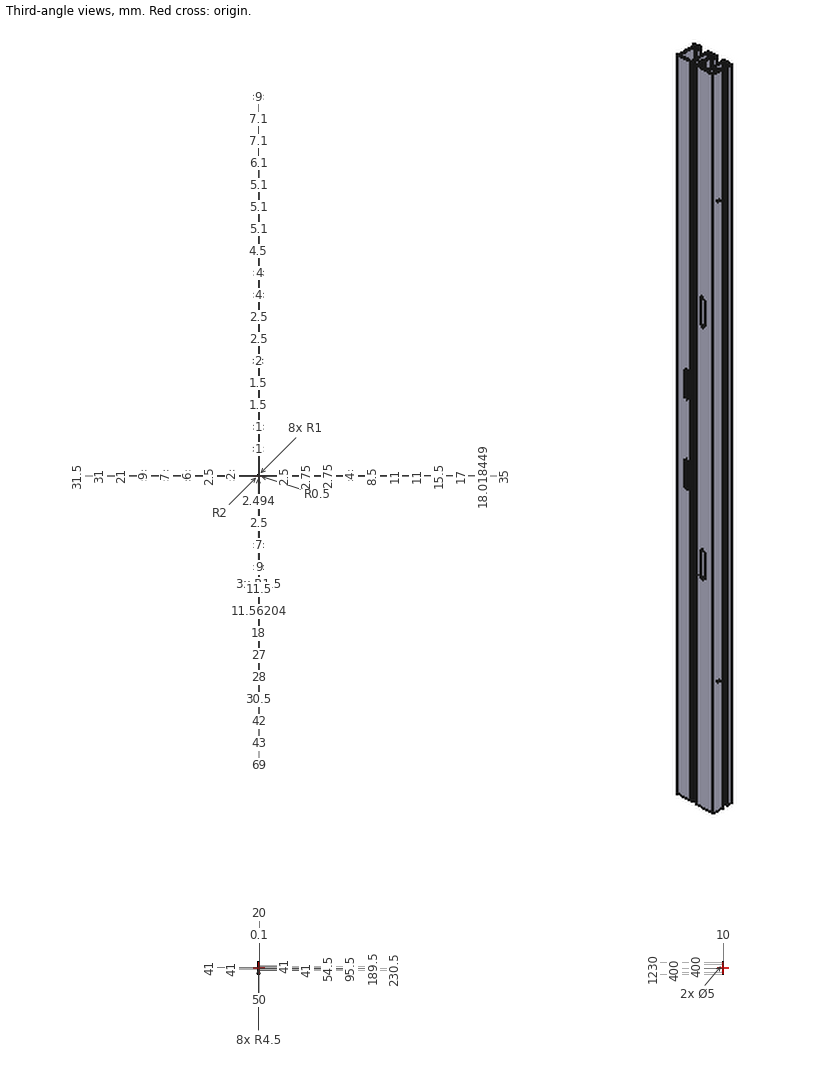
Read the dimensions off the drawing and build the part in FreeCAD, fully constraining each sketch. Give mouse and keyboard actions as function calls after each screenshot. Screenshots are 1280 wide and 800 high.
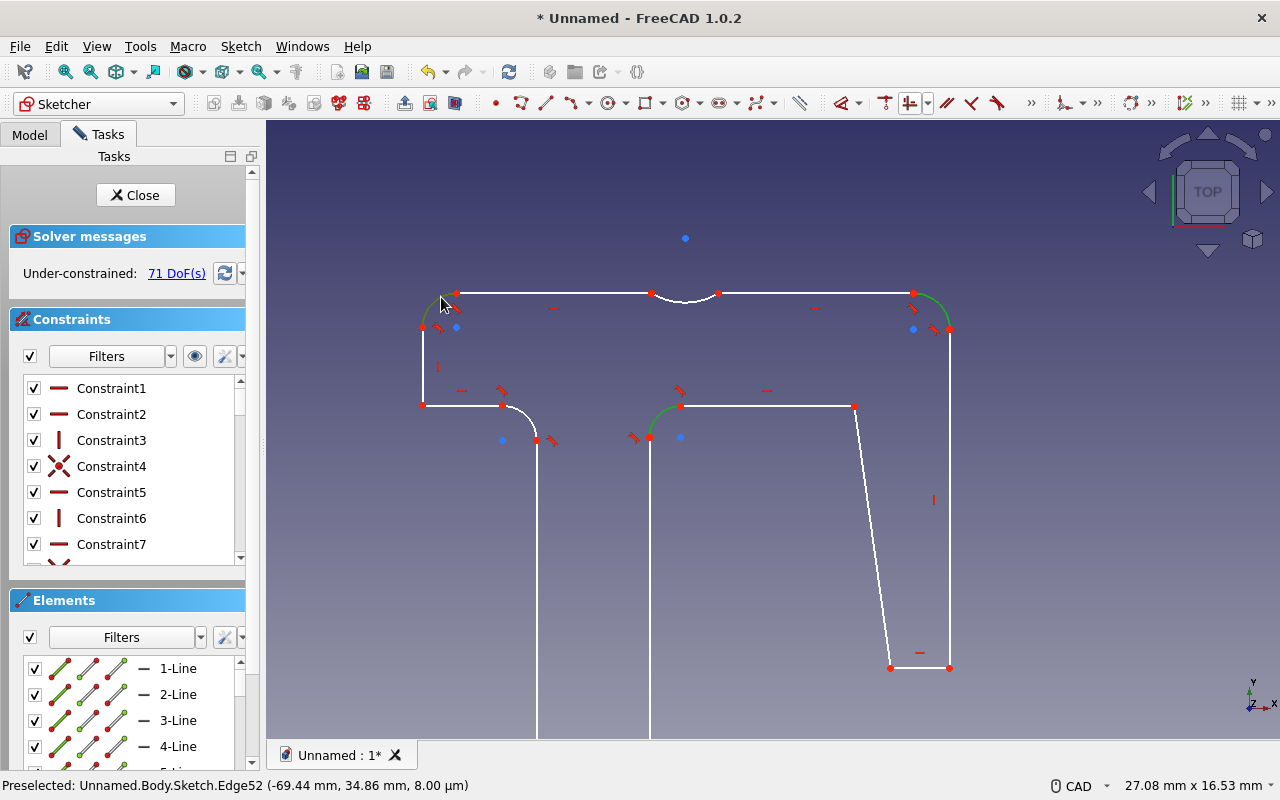
click(533, 425)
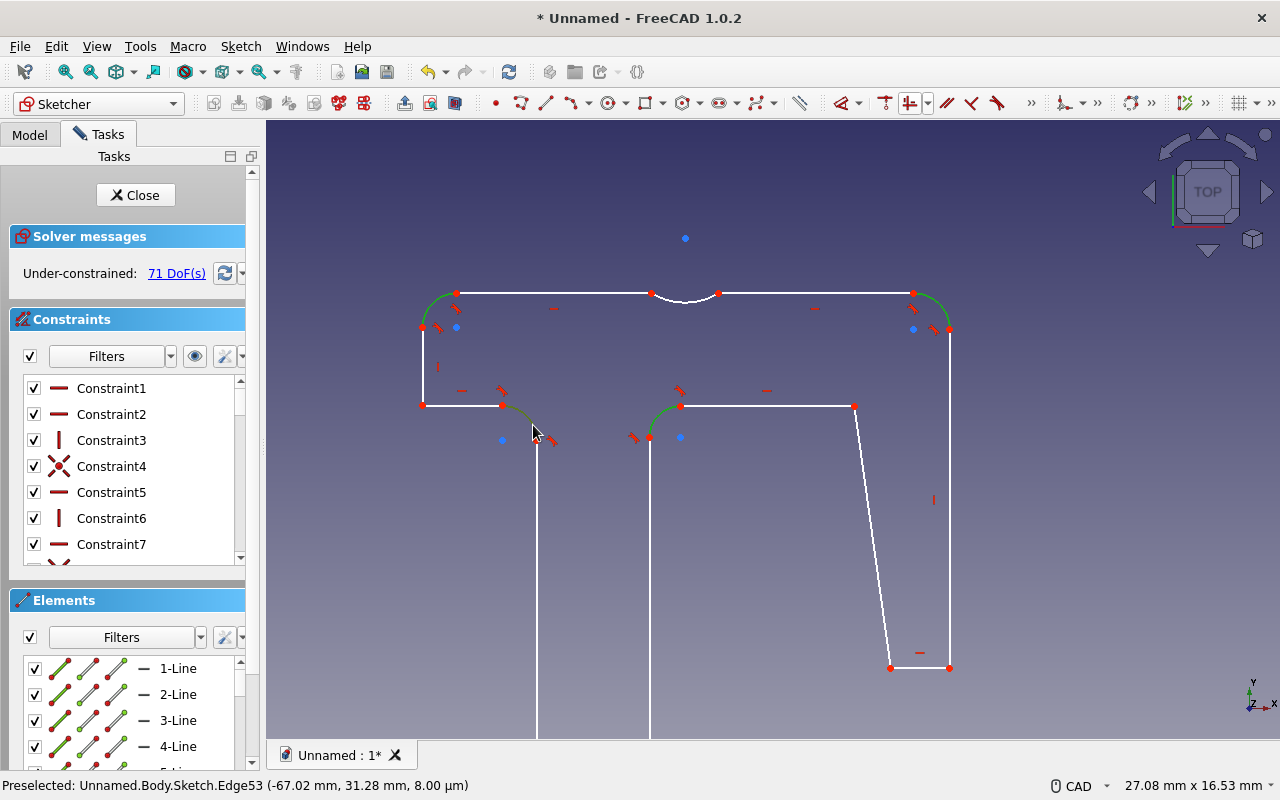
scroll(444, 299, down, 8)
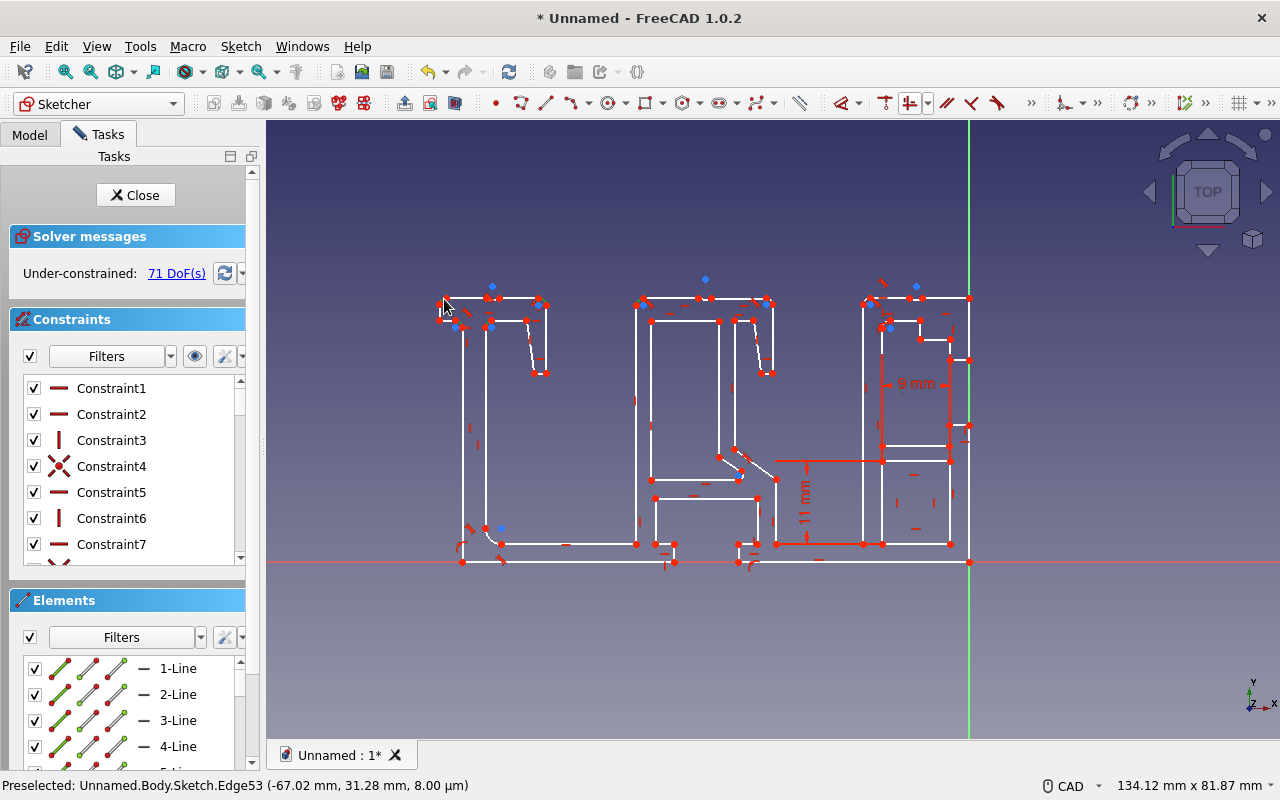
scroll(886, 322, up, 7)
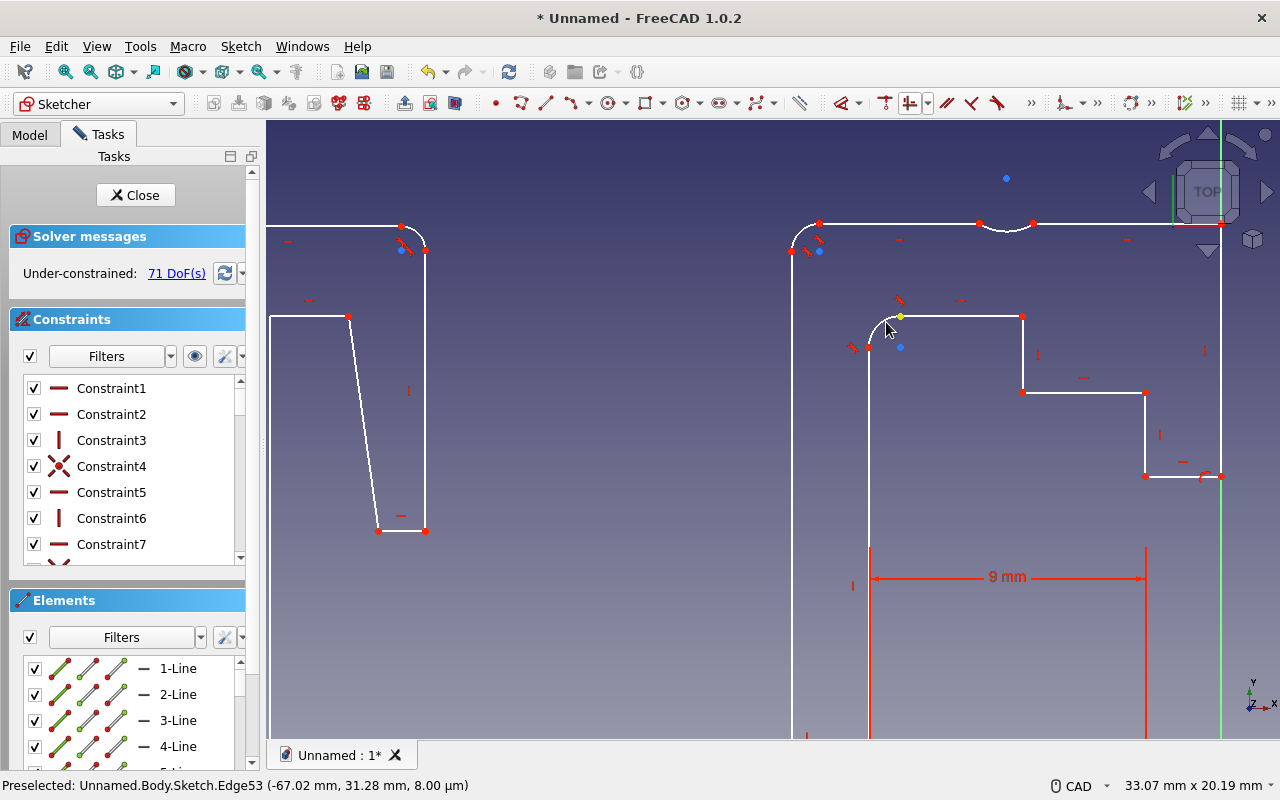
click(886, 320)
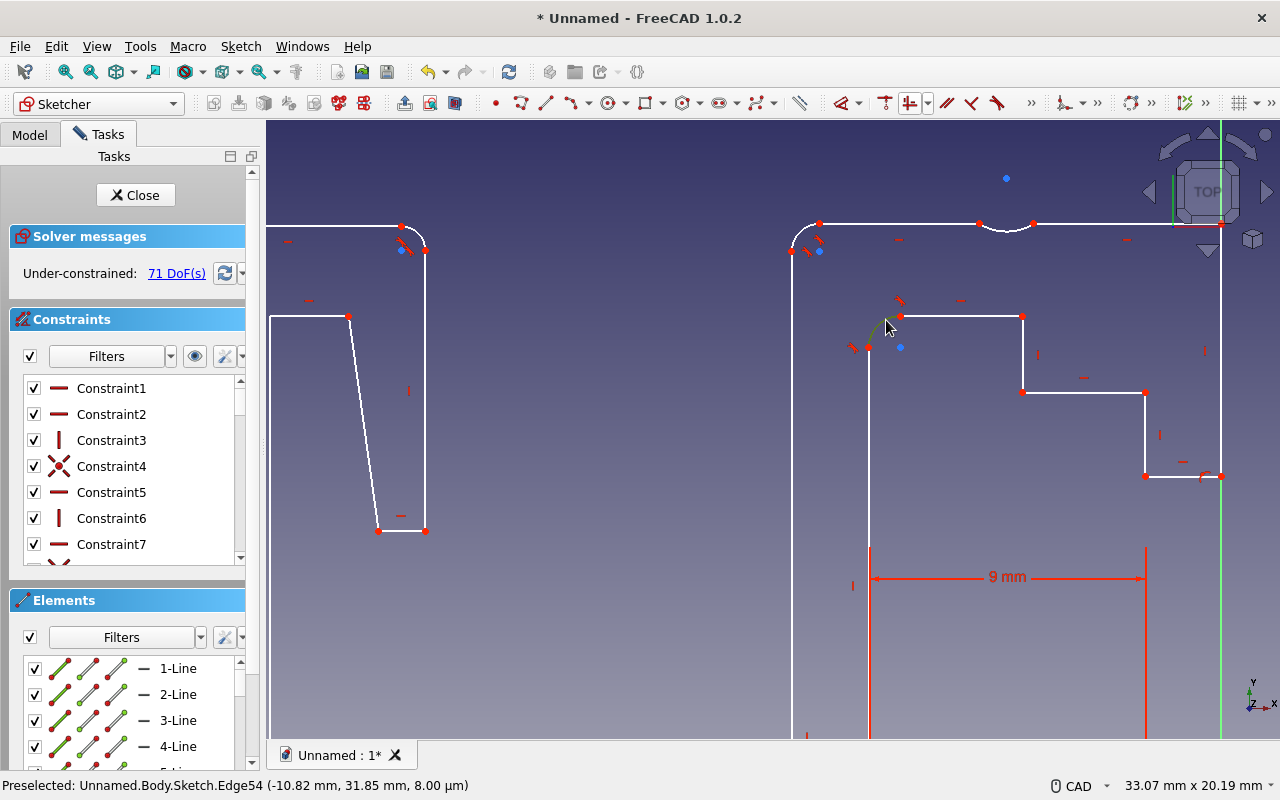
click(807, 227)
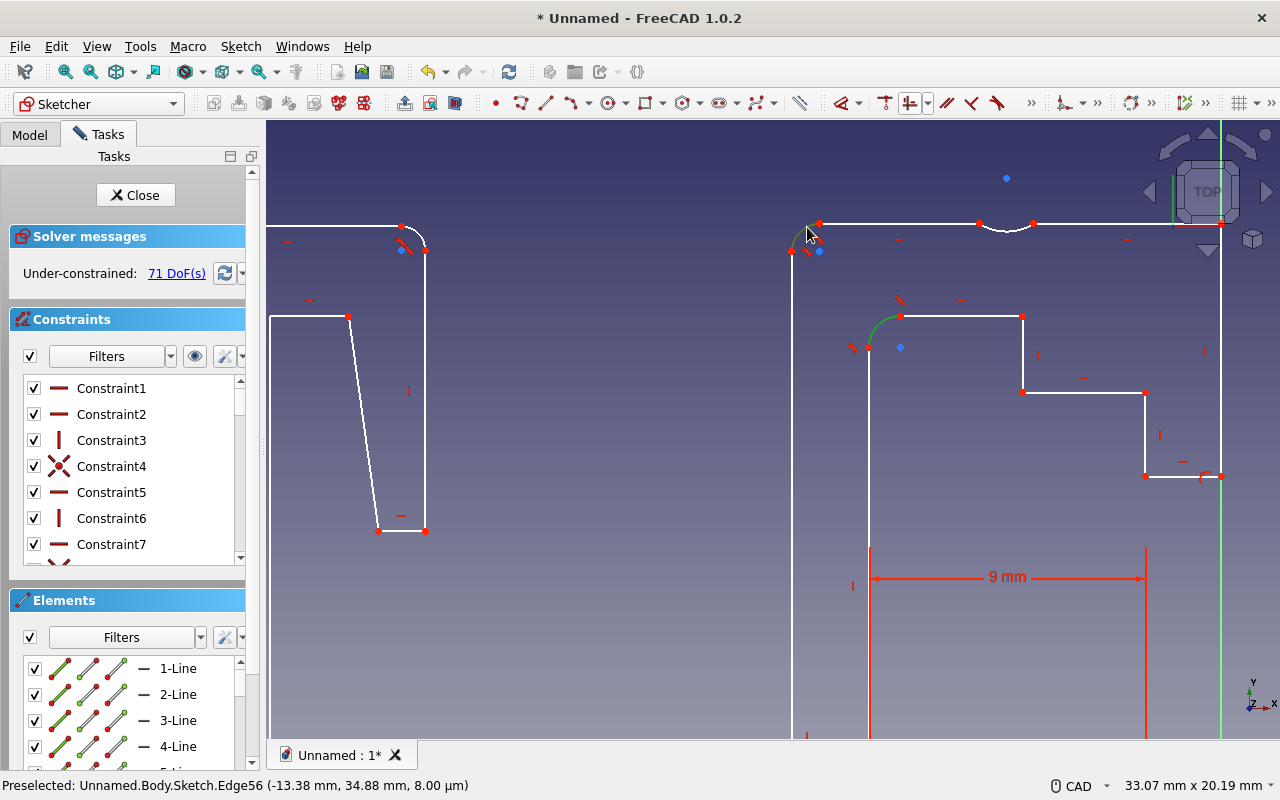
scroll(423, 239, up, 2)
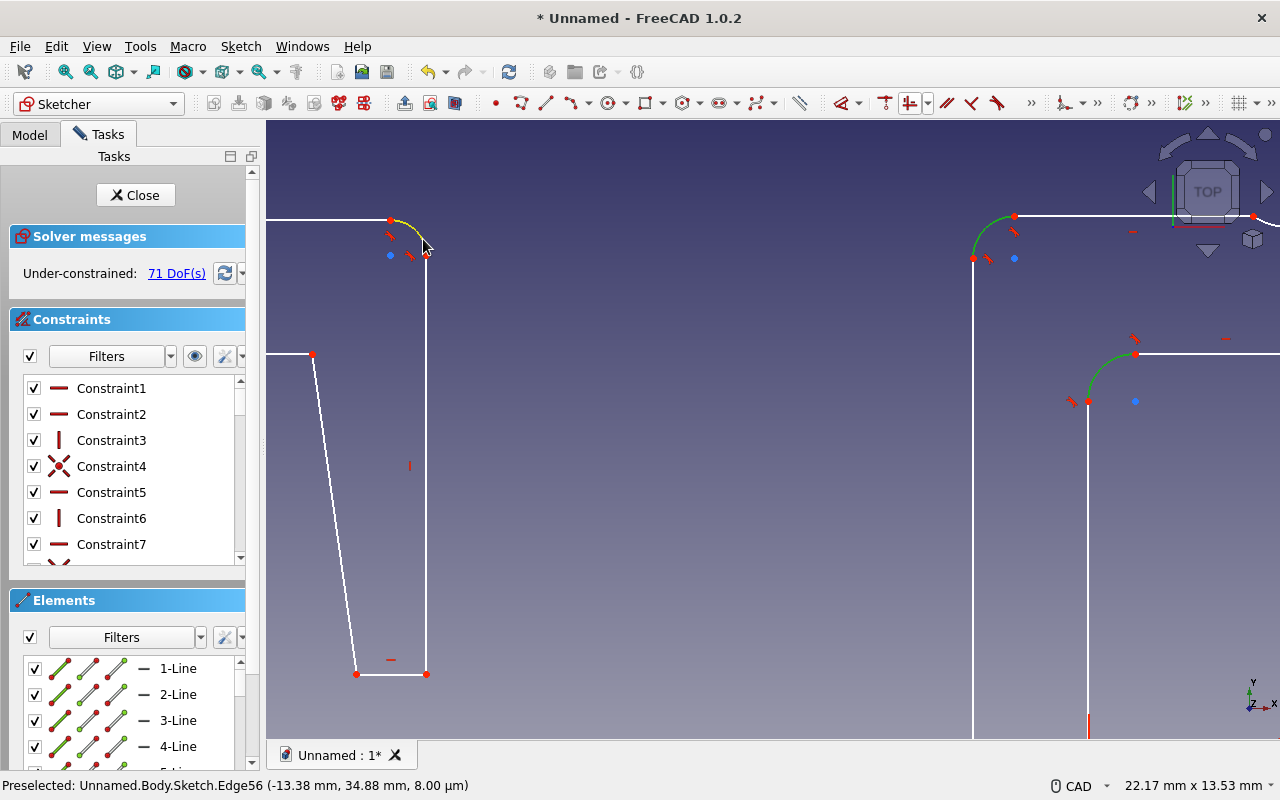
click(422, 239)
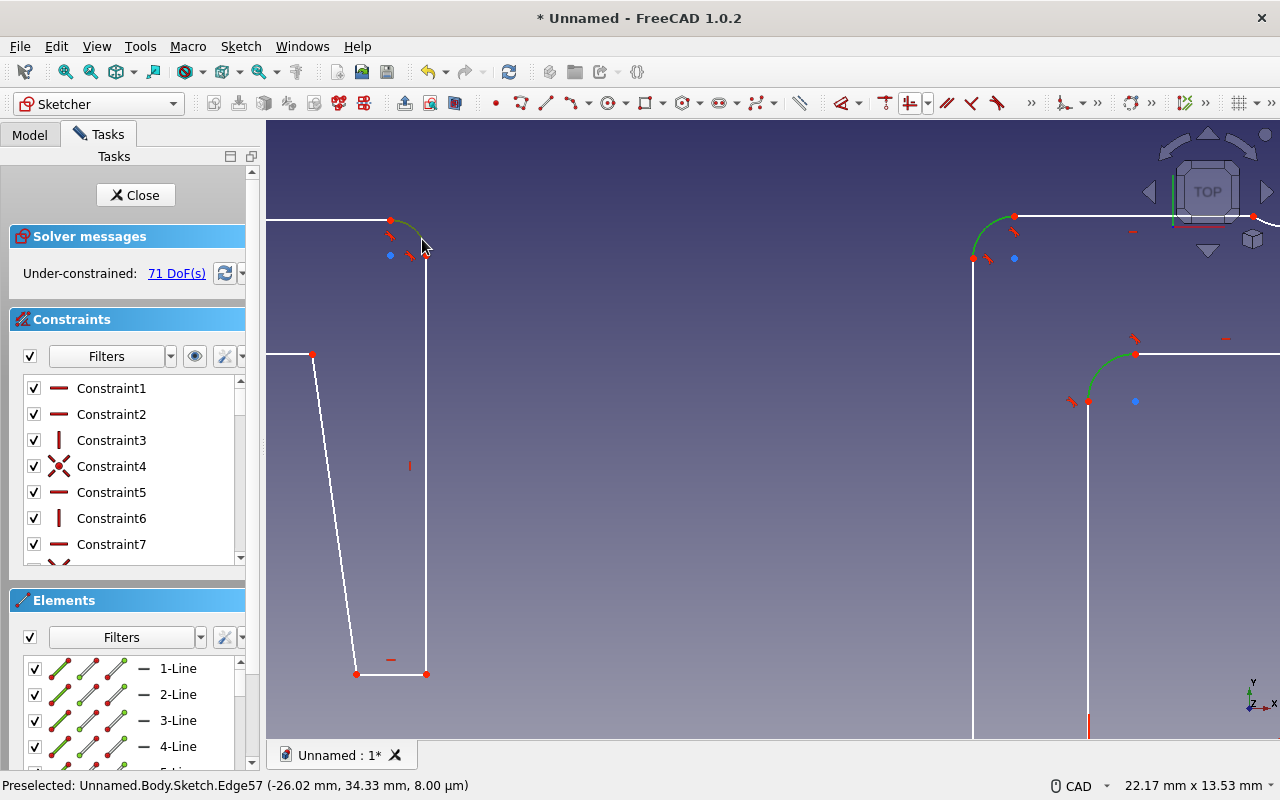
key(e)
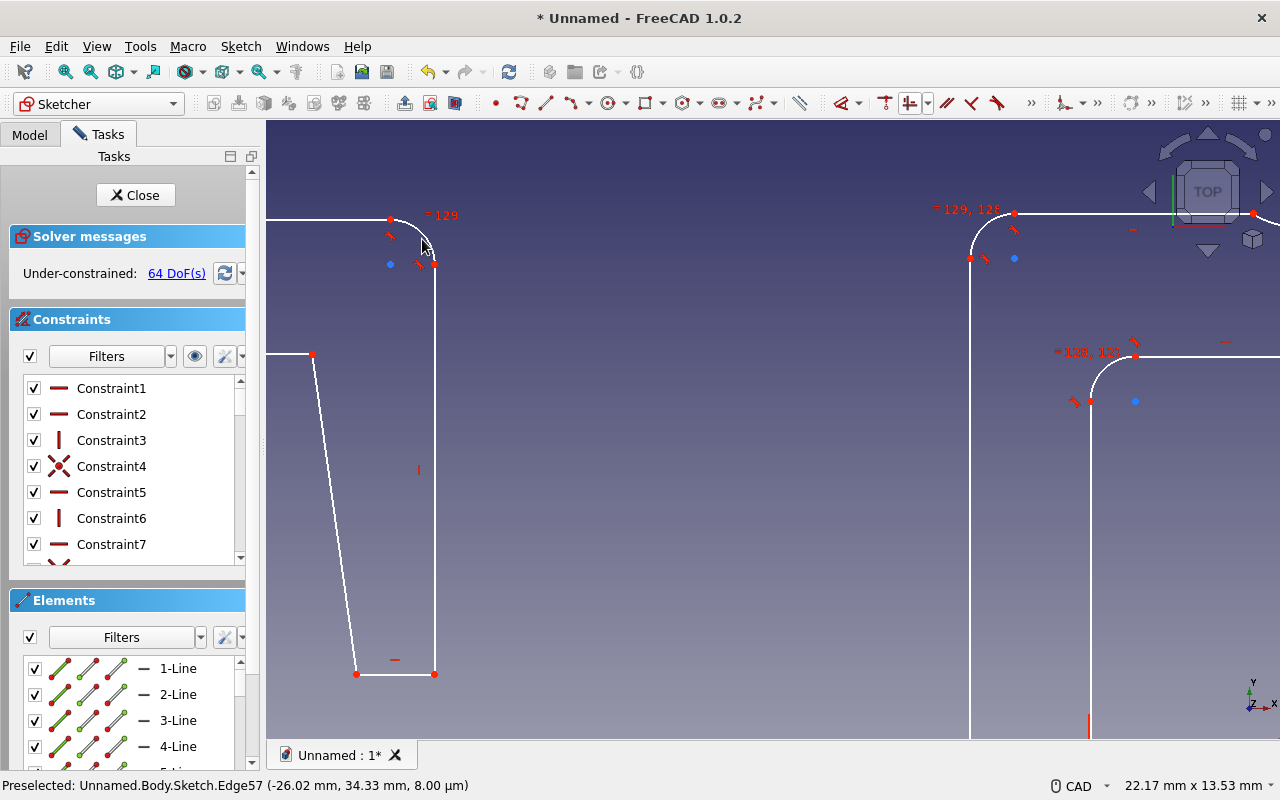
scroll(841, 314, down, 9)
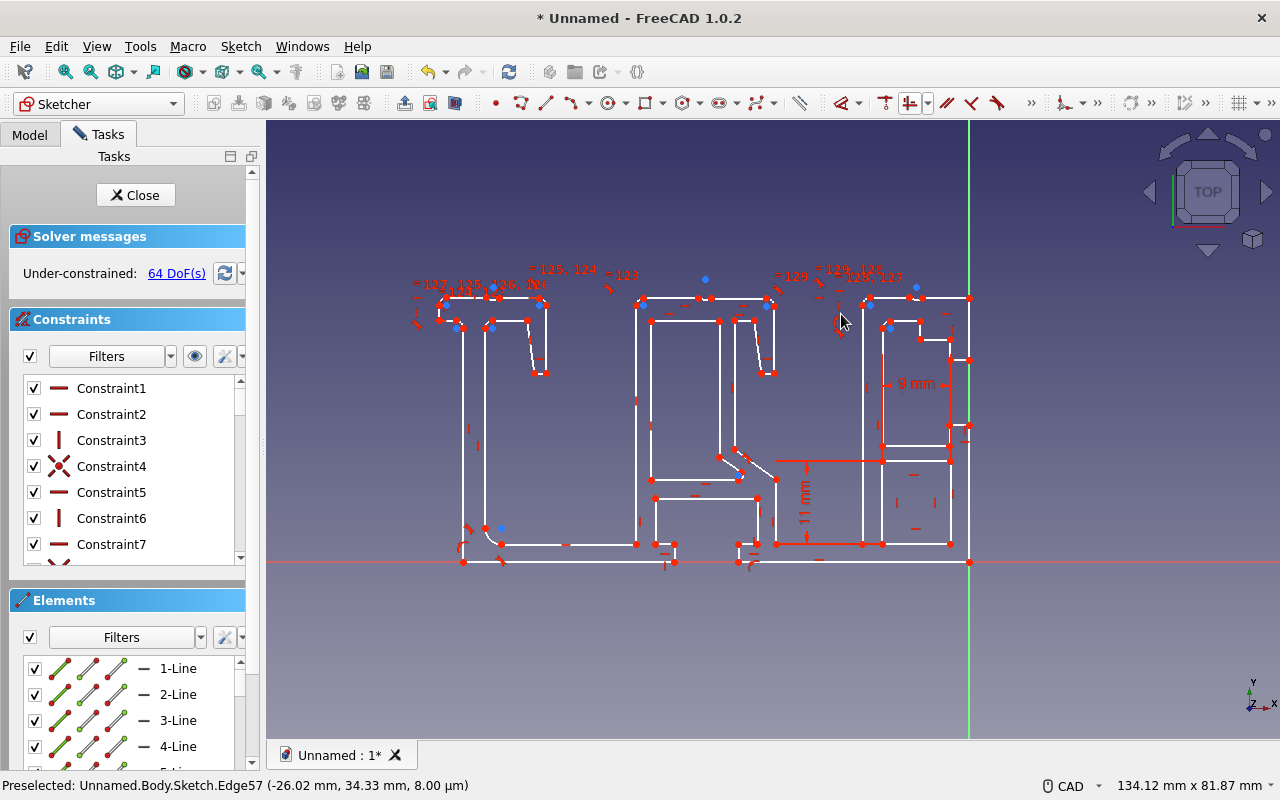
scroll(702, 299, up, 7)